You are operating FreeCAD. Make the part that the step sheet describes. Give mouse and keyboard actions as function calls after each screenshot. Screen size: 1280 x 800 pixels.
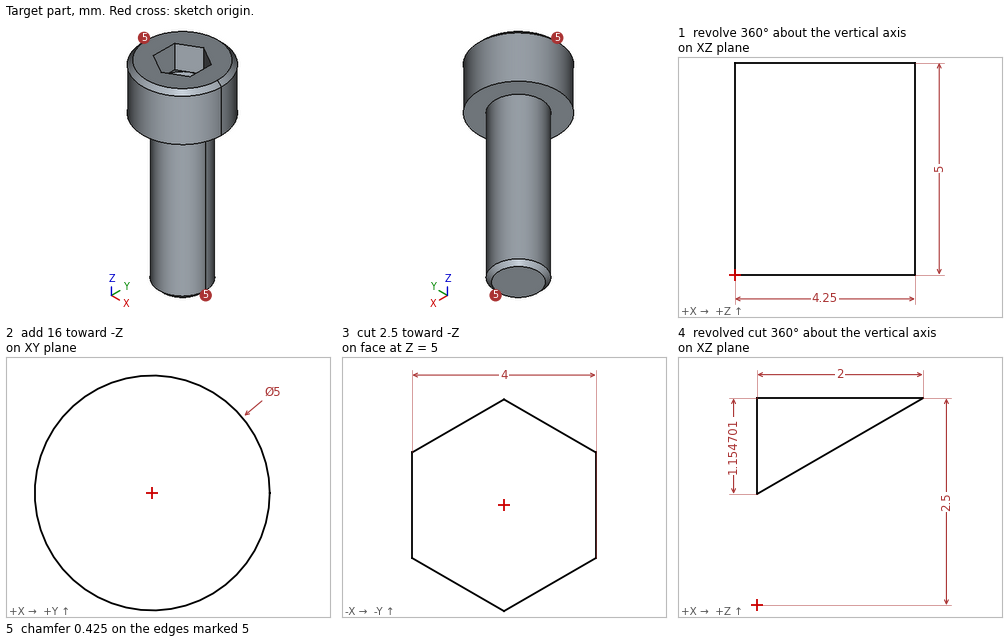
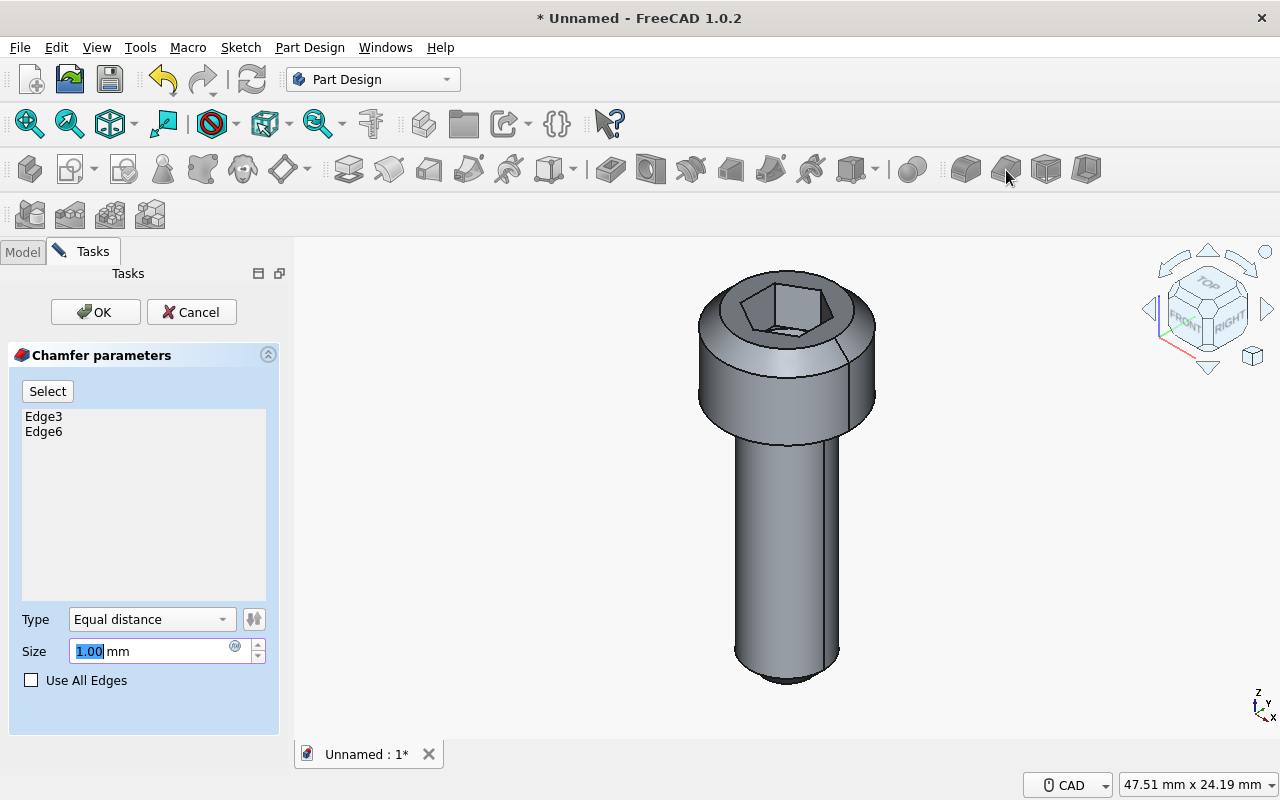
text(0.425)
key(Tab)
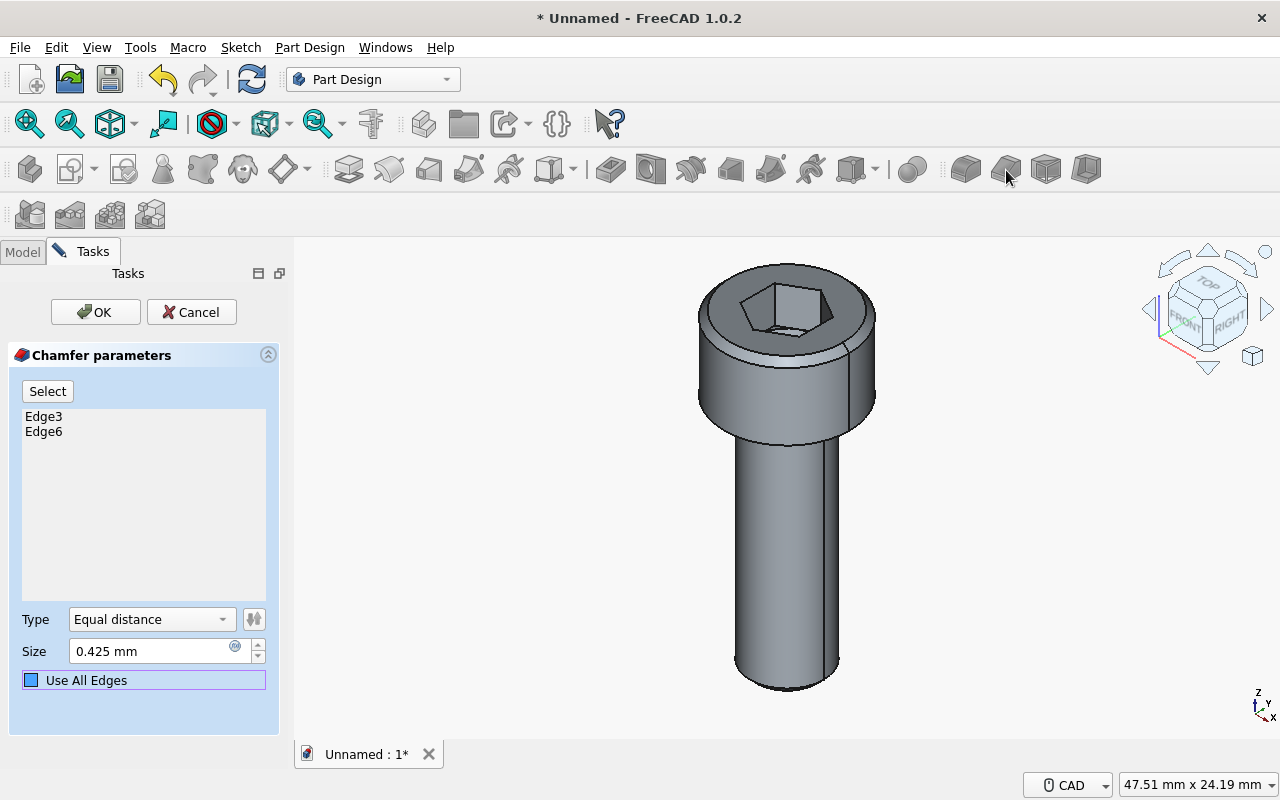
click(96, 312)